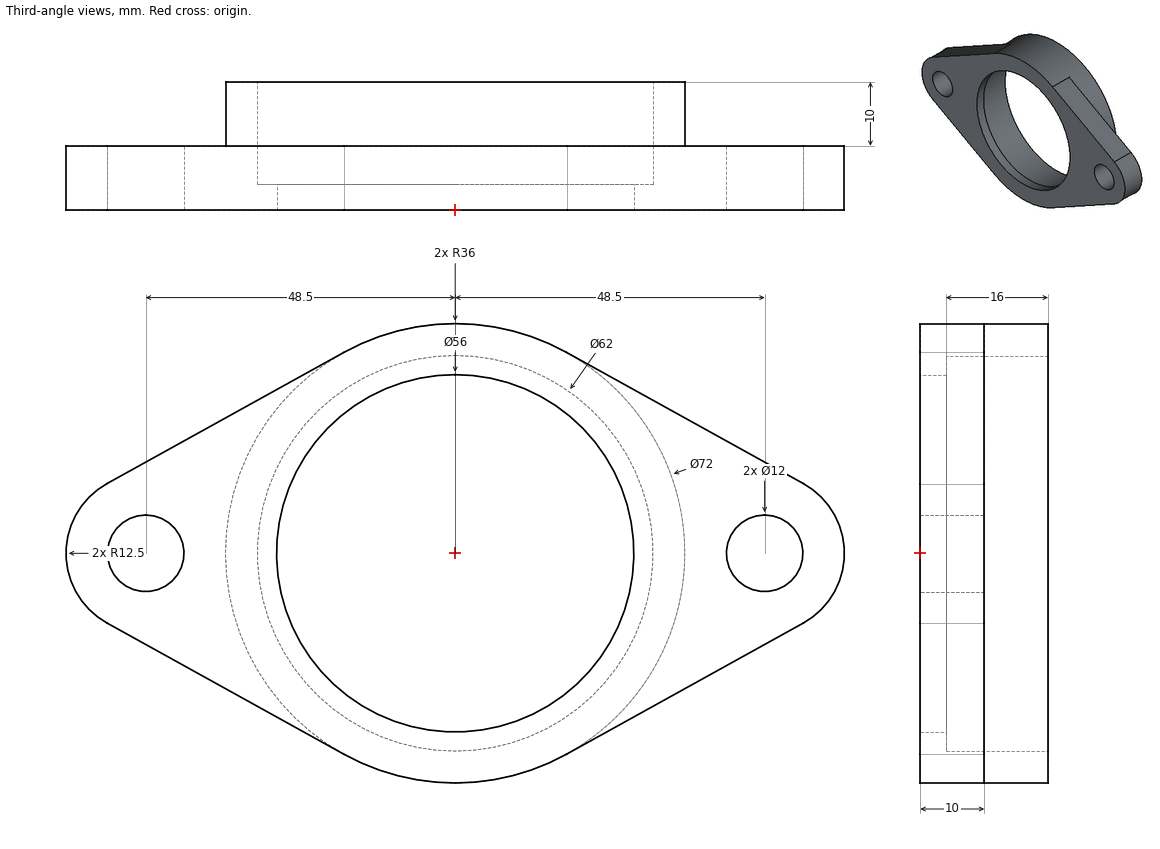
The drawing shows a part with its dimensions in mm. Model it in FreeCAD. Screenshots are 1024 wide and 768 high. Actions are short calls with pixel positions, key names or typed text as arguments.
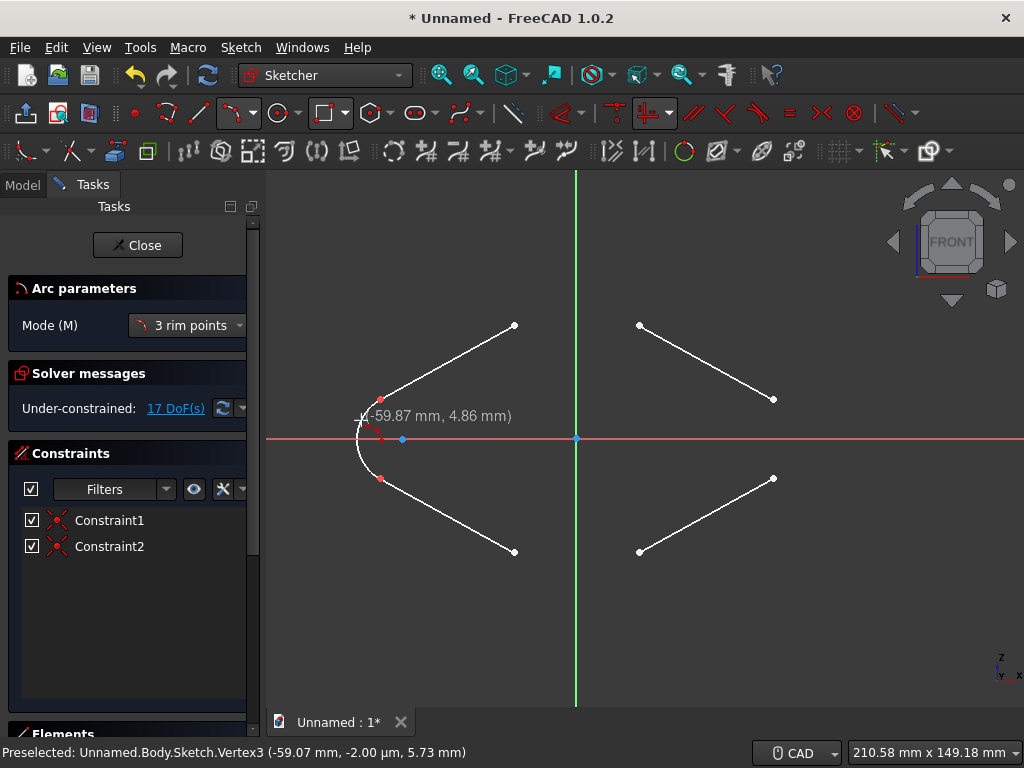
click(514, 326)
click(639, 326)
click(603, 312)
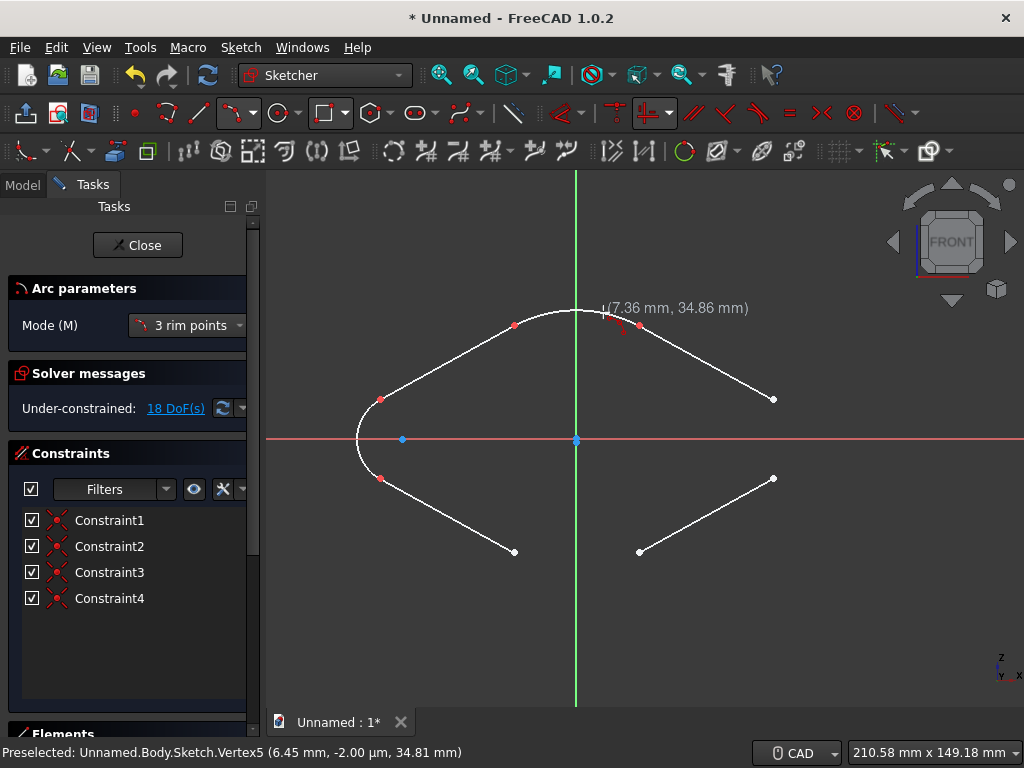
click(773, 400)
click(773, 479)
click(792, 457)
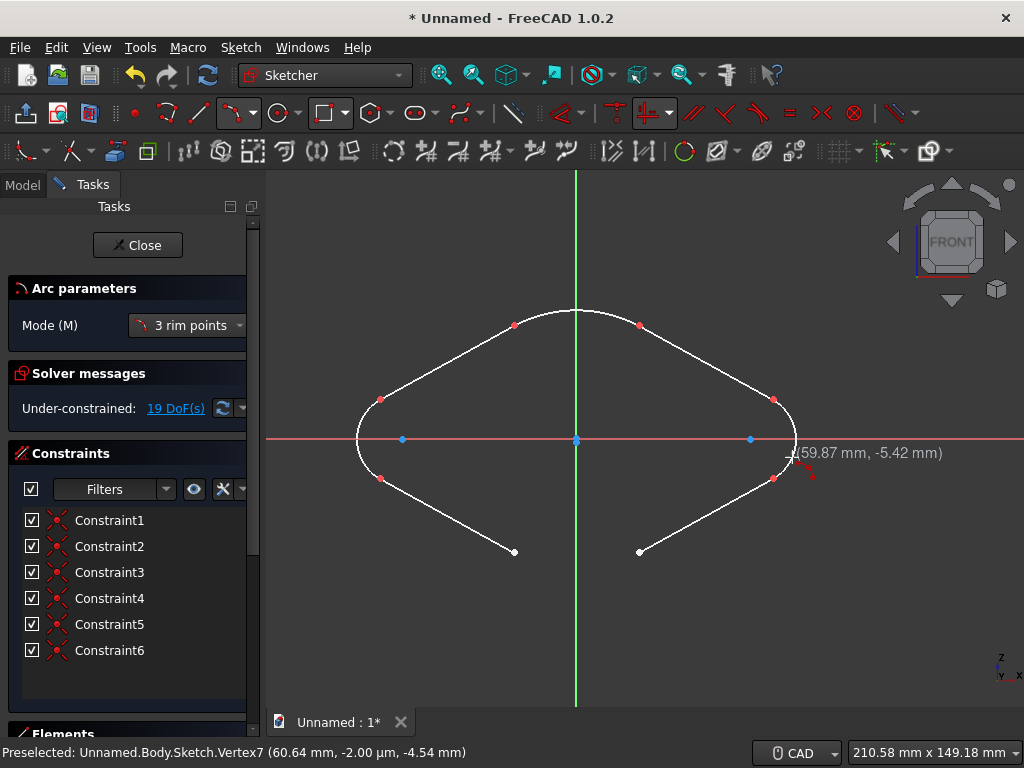
click(639, 553)
click(514, 553)
click(550, 565)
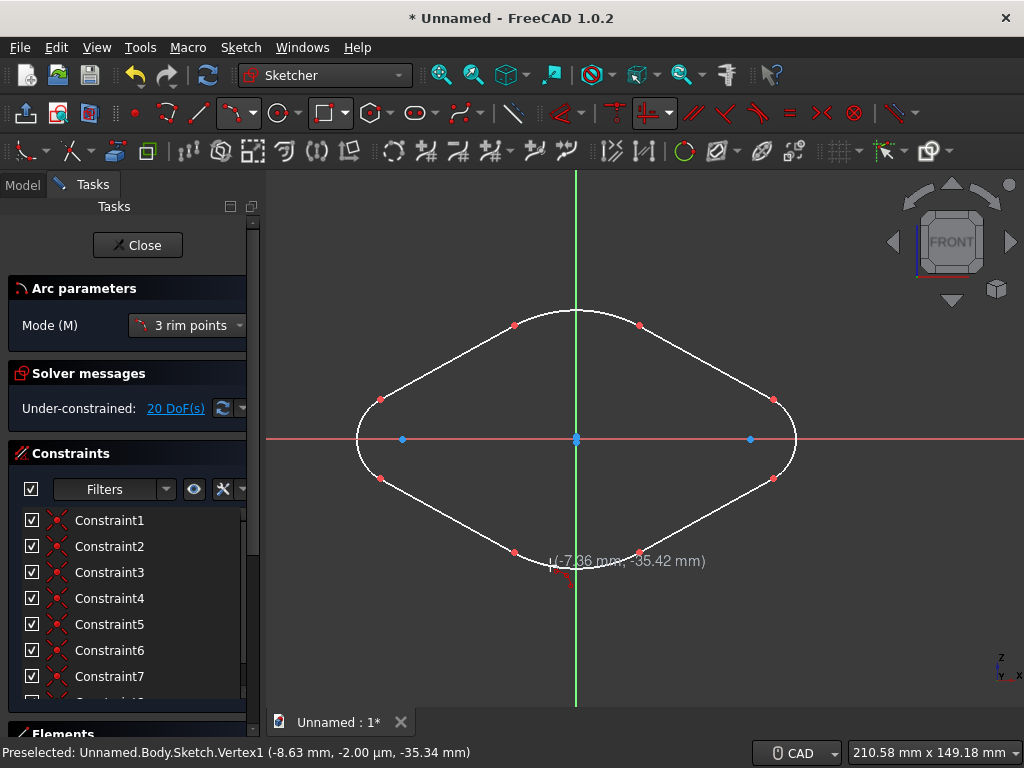
click(278, 114)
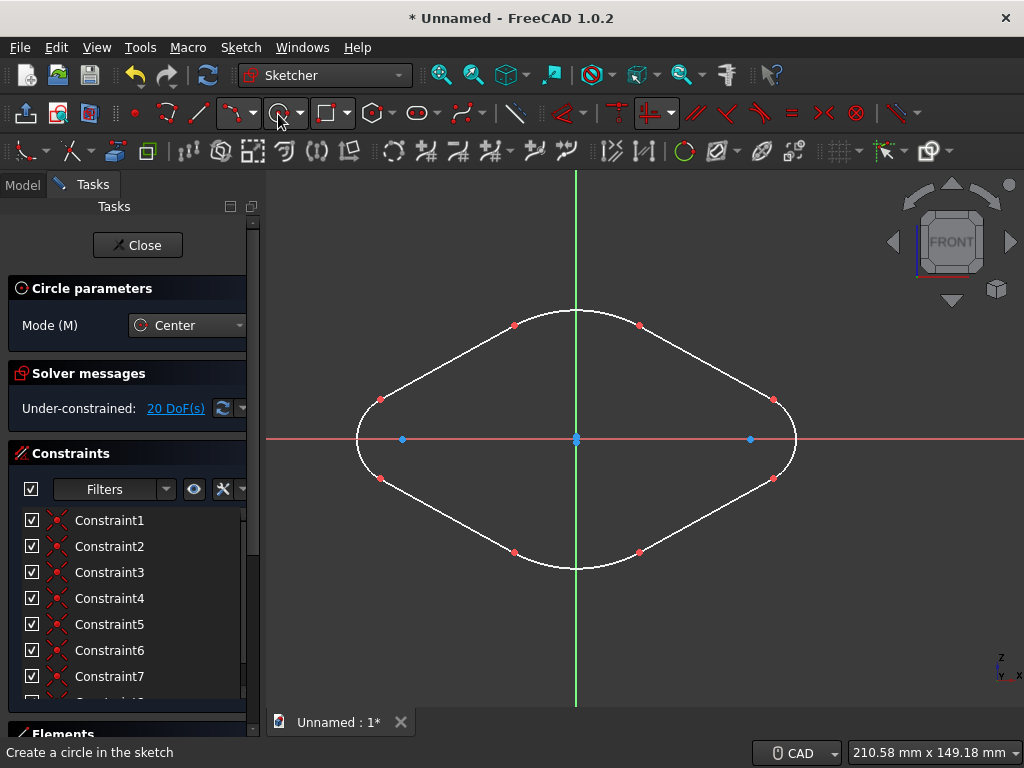
click(751, 438)
click(766, 423)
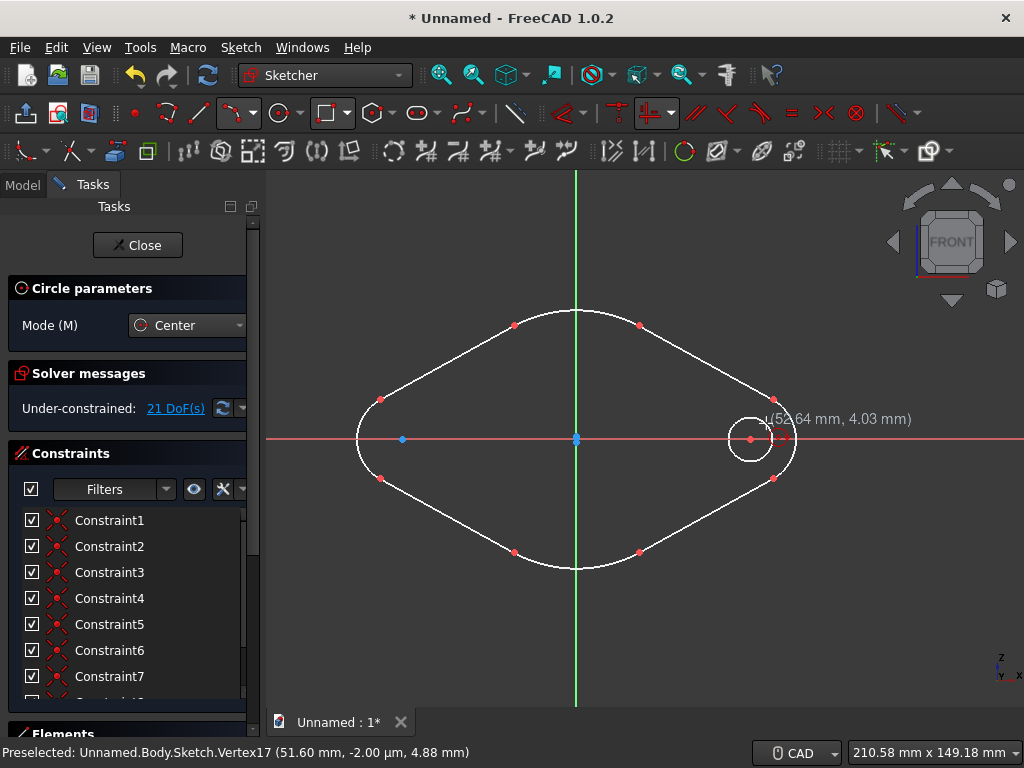
click(402, 438)
click(417, 423)
key(Escape)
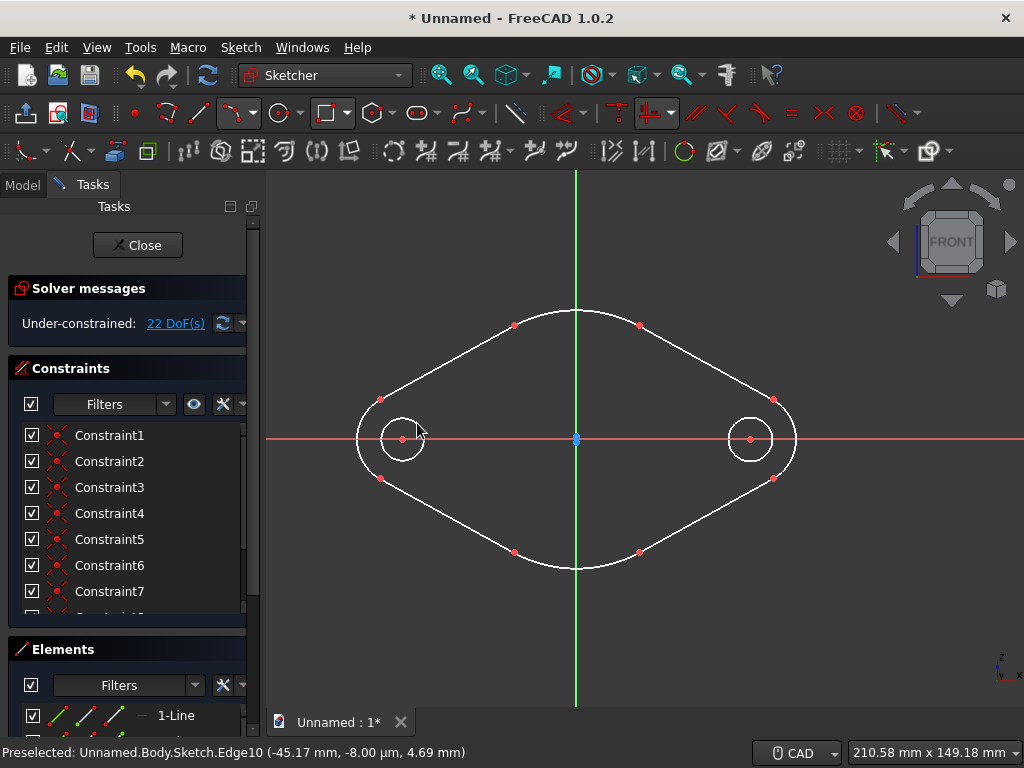
click(474, 531)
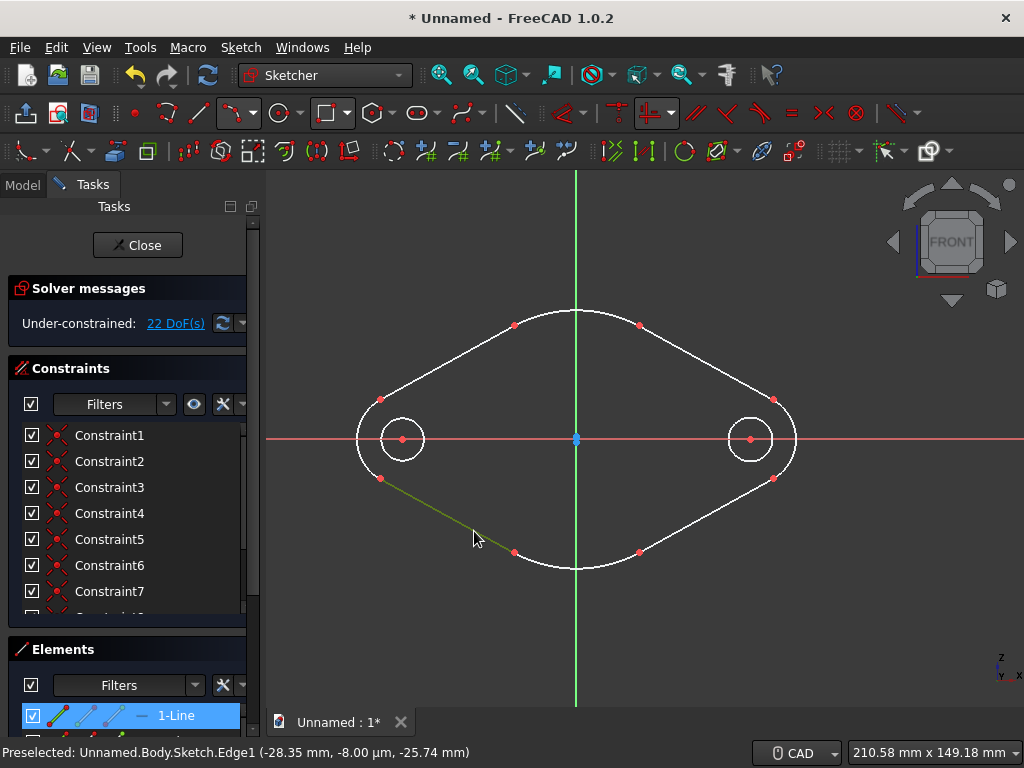
click(361, 421)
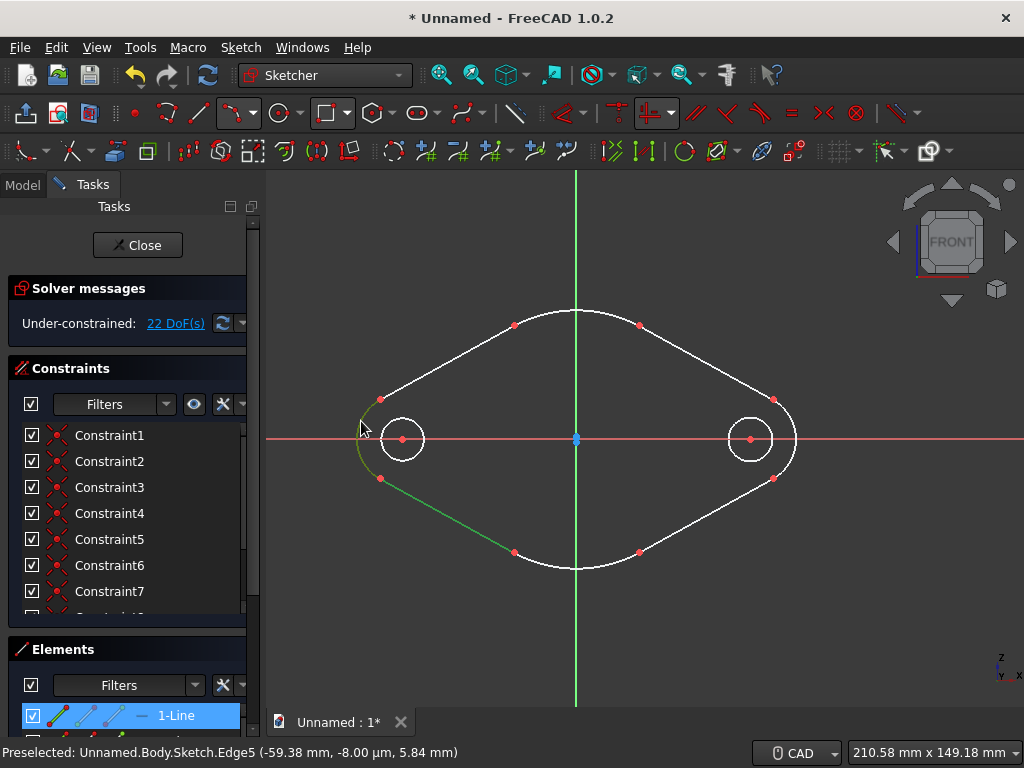
click(760, 114)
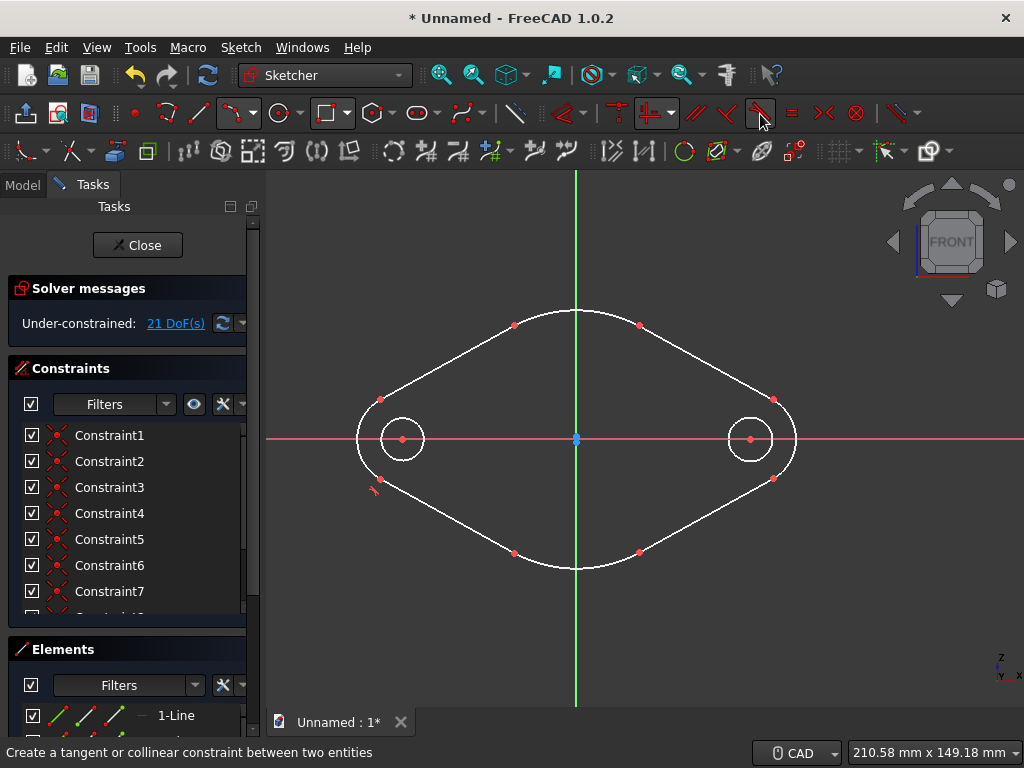
click(474, 531)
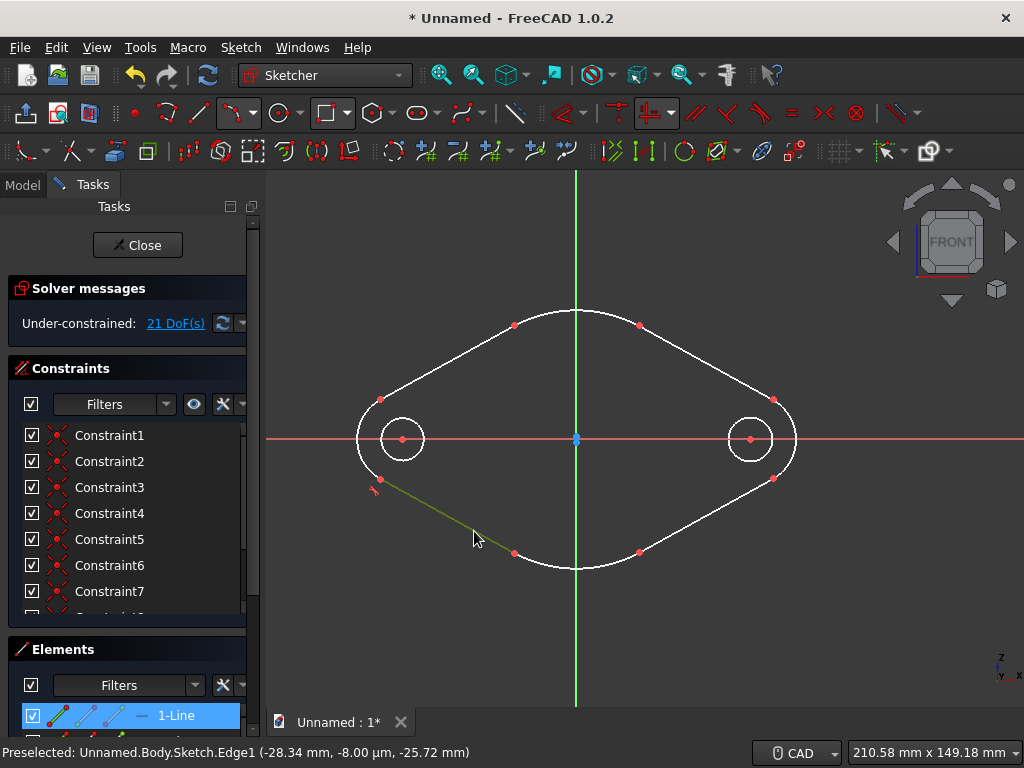
click(551, 566)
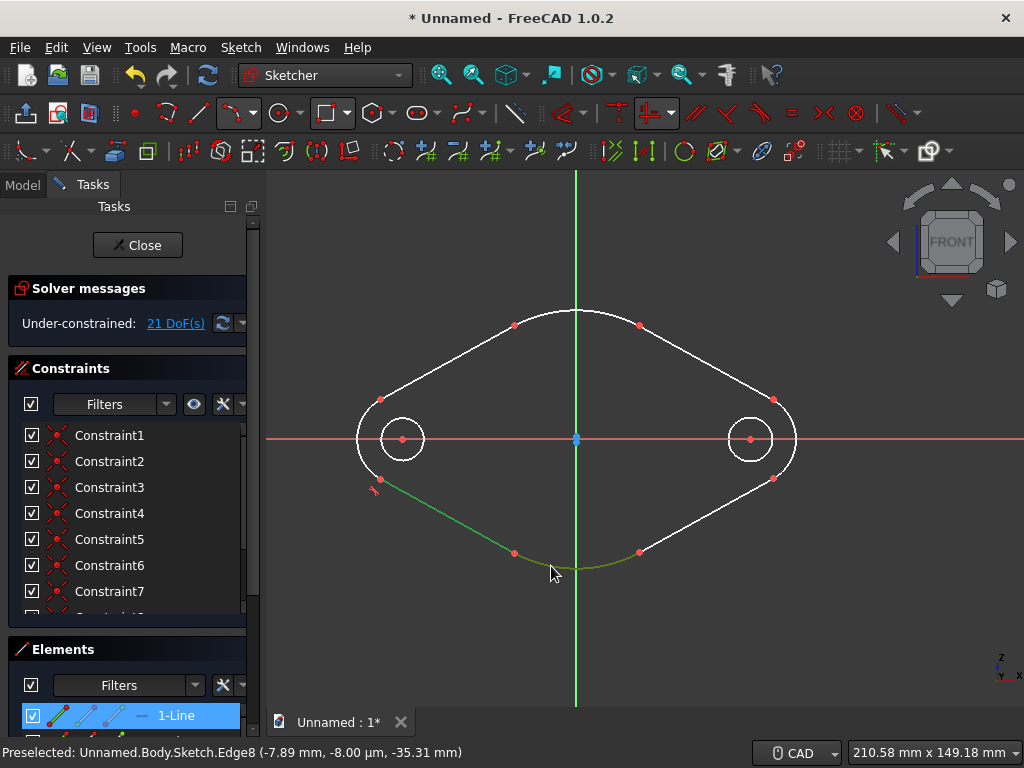
click(760, 114)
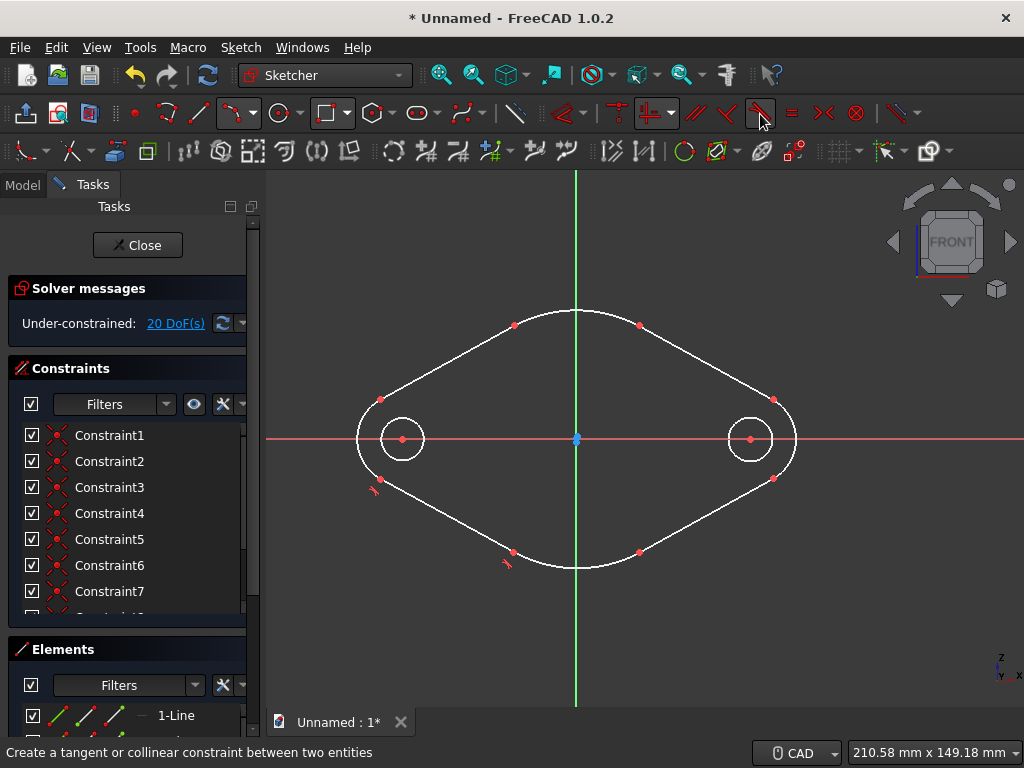
click(420, 378)